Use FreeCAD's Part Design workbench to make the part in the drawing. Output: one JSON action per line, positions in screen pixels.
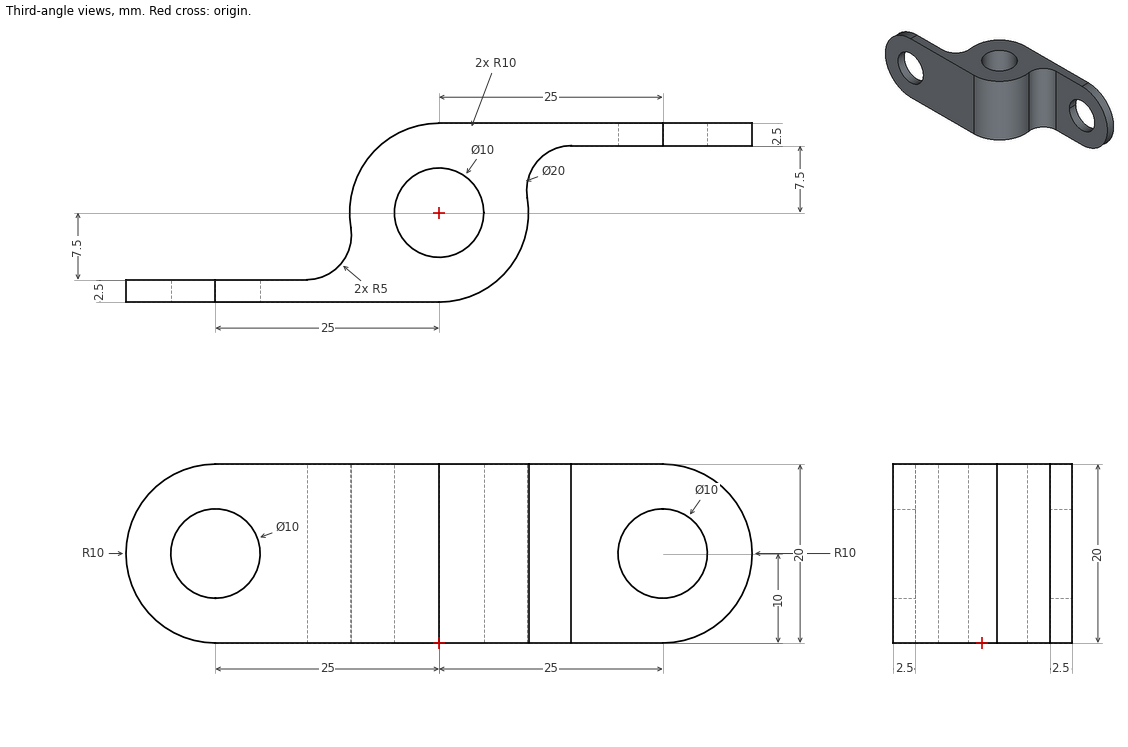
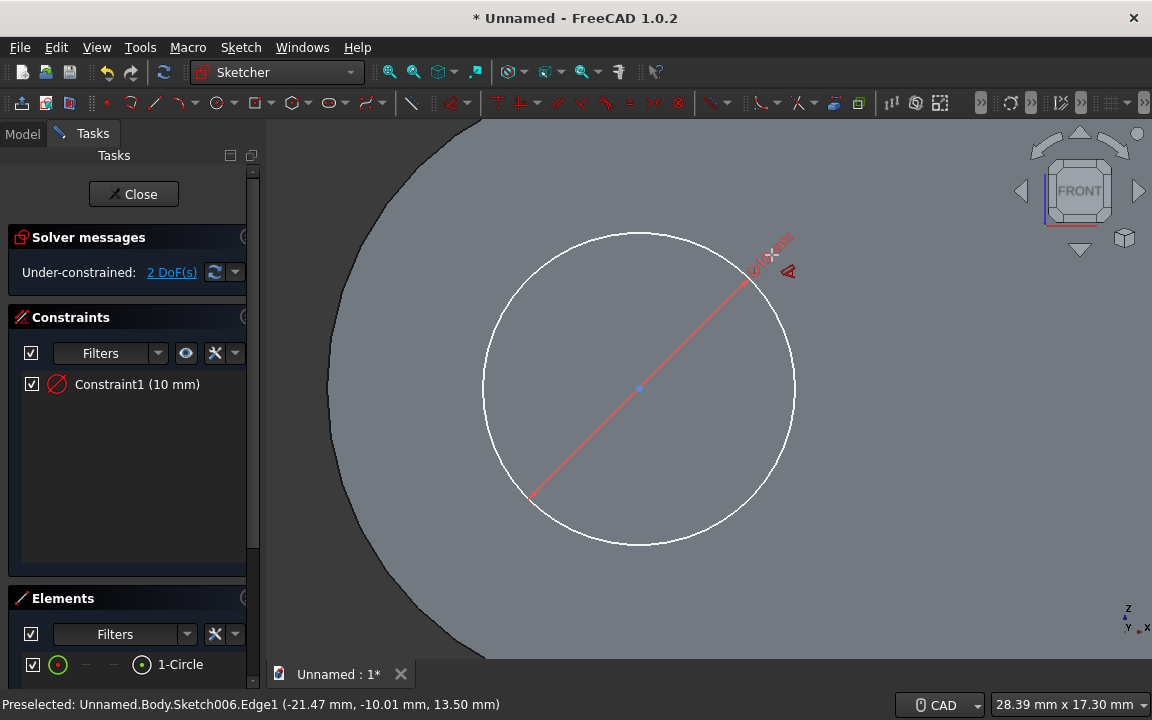
{"action": "left_click", "coordinate": [639, 389]}
{"action": "left_click", "coordinate": [813, 355]}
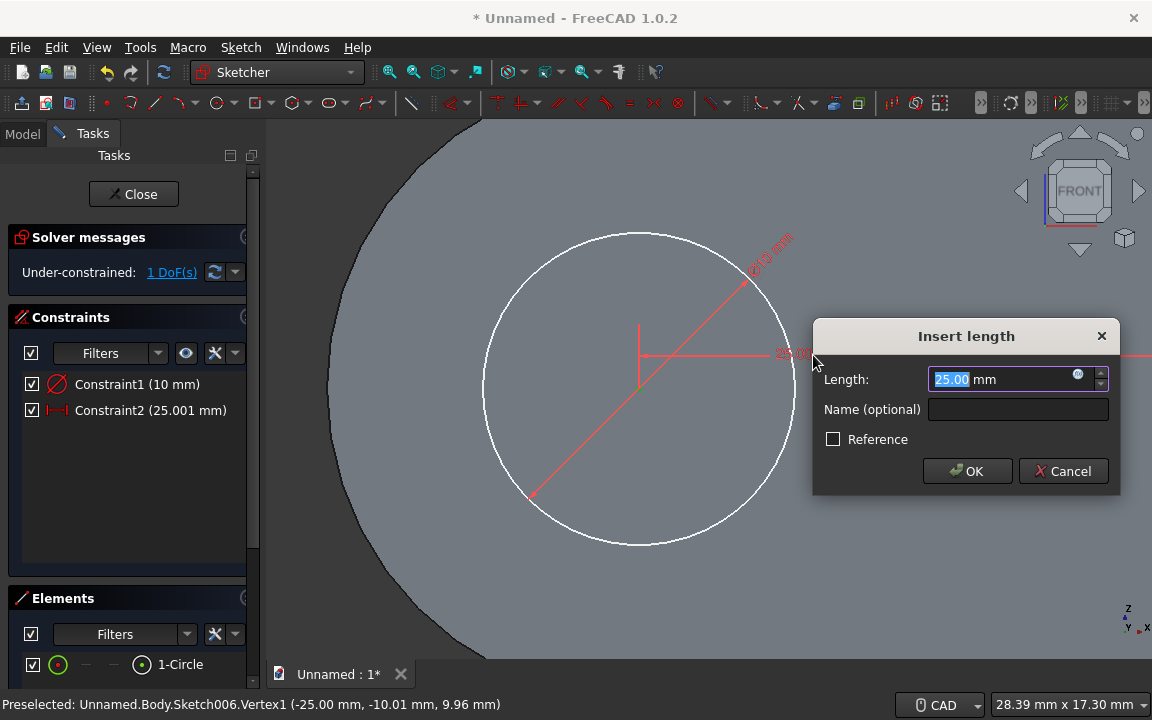
{"action": "type", "text": "25"}
{"action": "key", "text": "Return"}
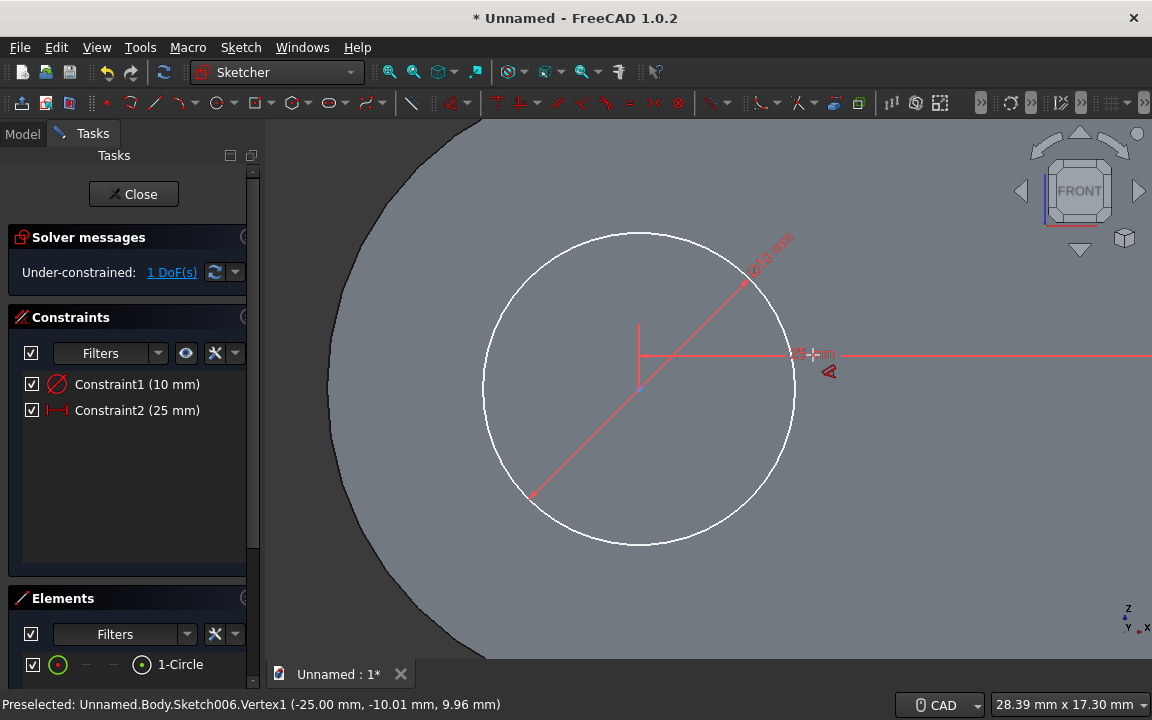
{"action": "left_click", "coordinate": [639, 389]}
{"action": "left_click", "coordinate": [605, 510]}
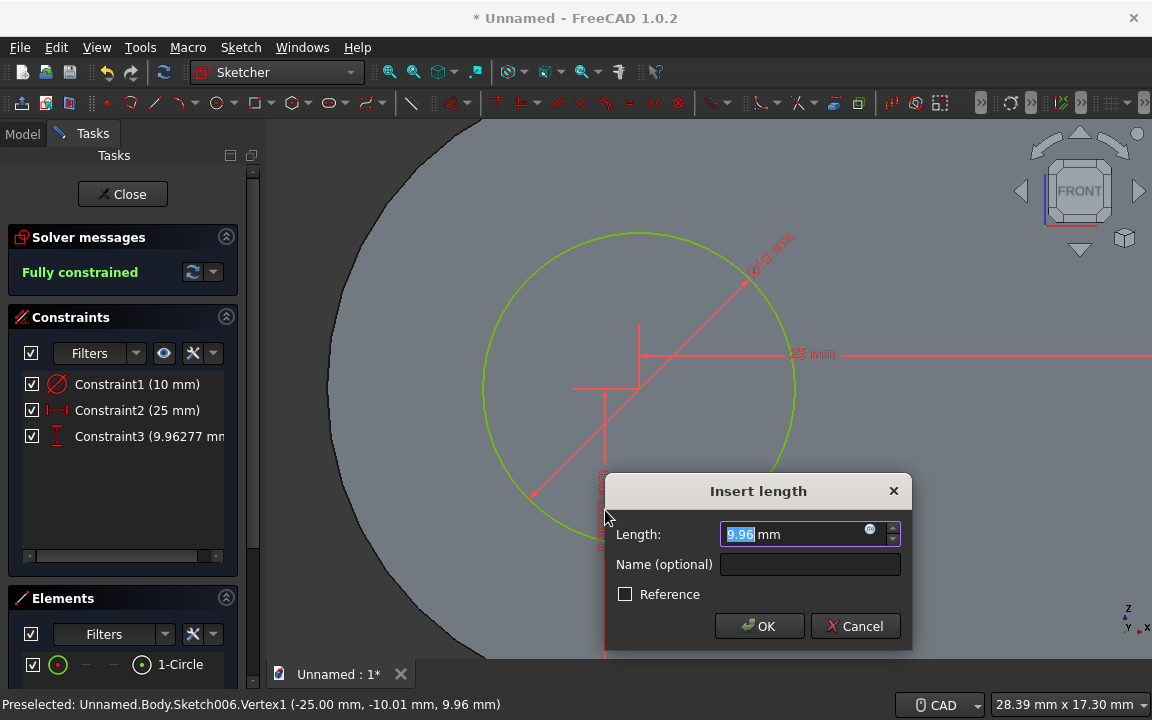
{"action": "type", "text": "10"}
{"action": "key", "text": "Return"}
{"action": "key", "text": "Escape"}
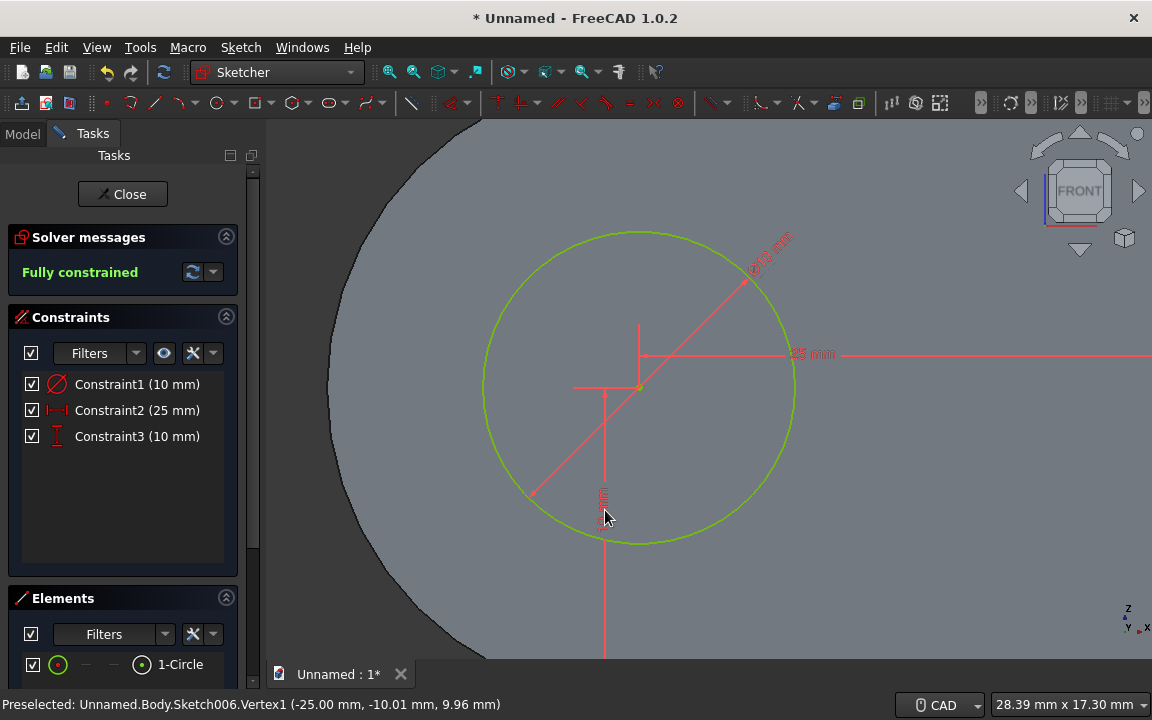
{"action": "left_click", "coordinate": [123, 194]}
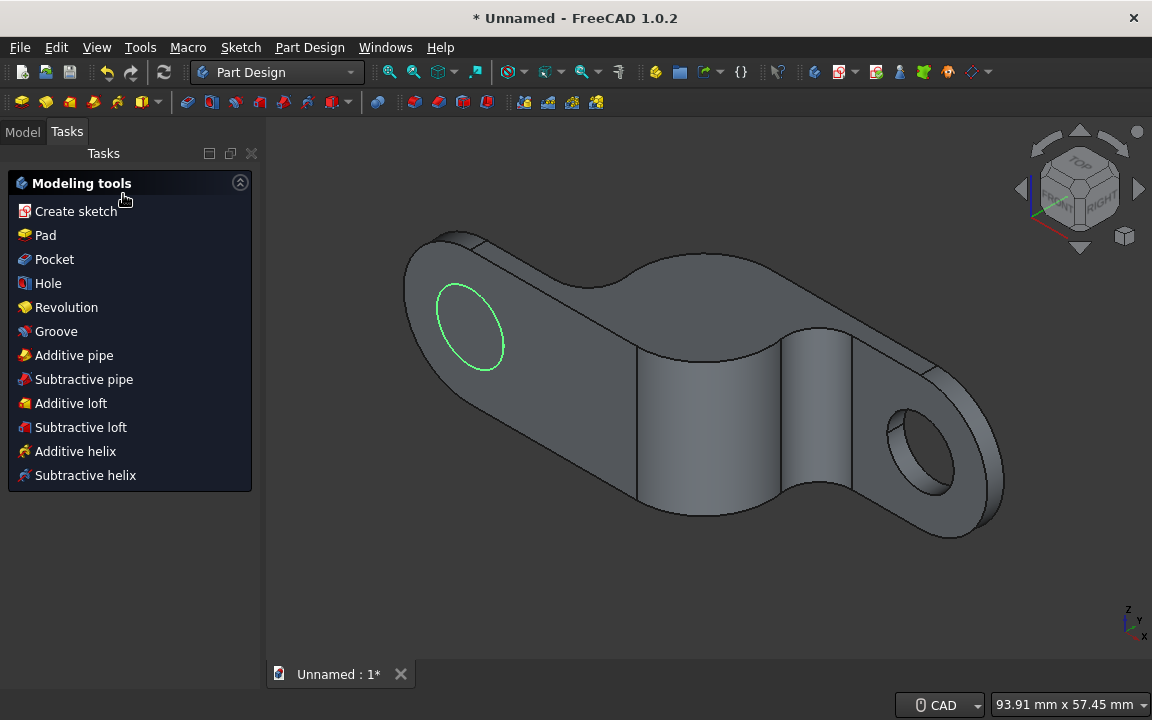
{"action": "left_click", "coordinate": [188, 102]}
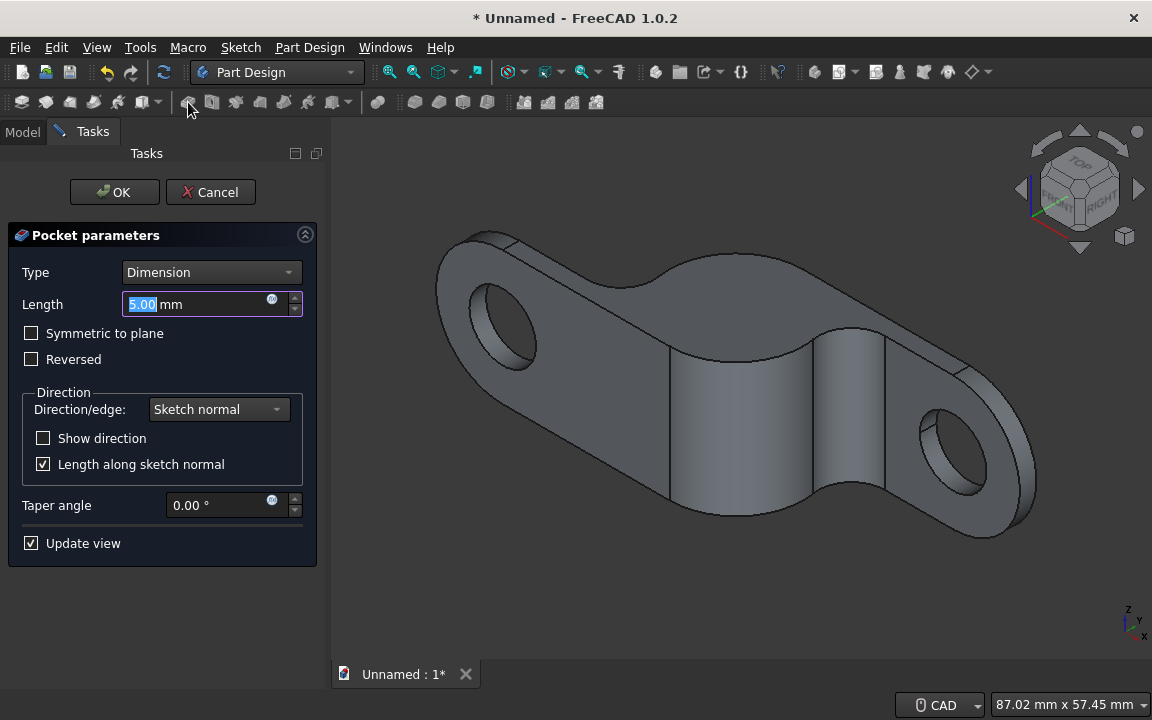
{"action": "type", "text": "2.5"}
{"action": "key", "text": "Tab"}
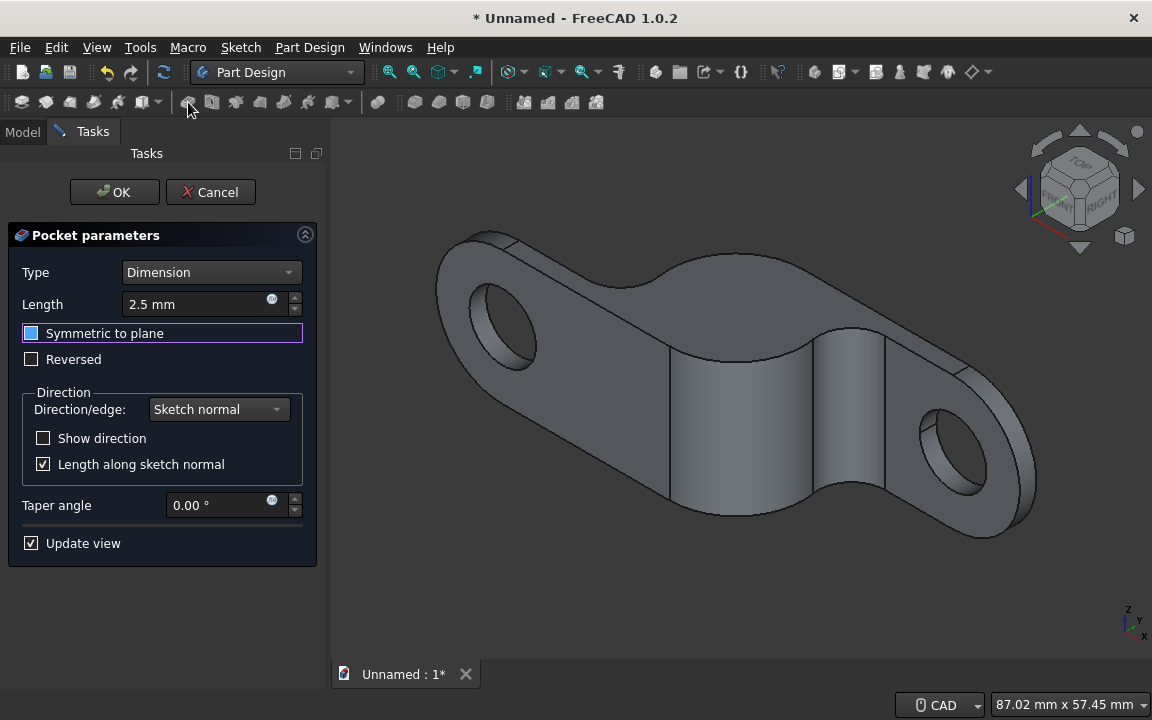
{"action": "left_click", "coordinate": [115, 192]}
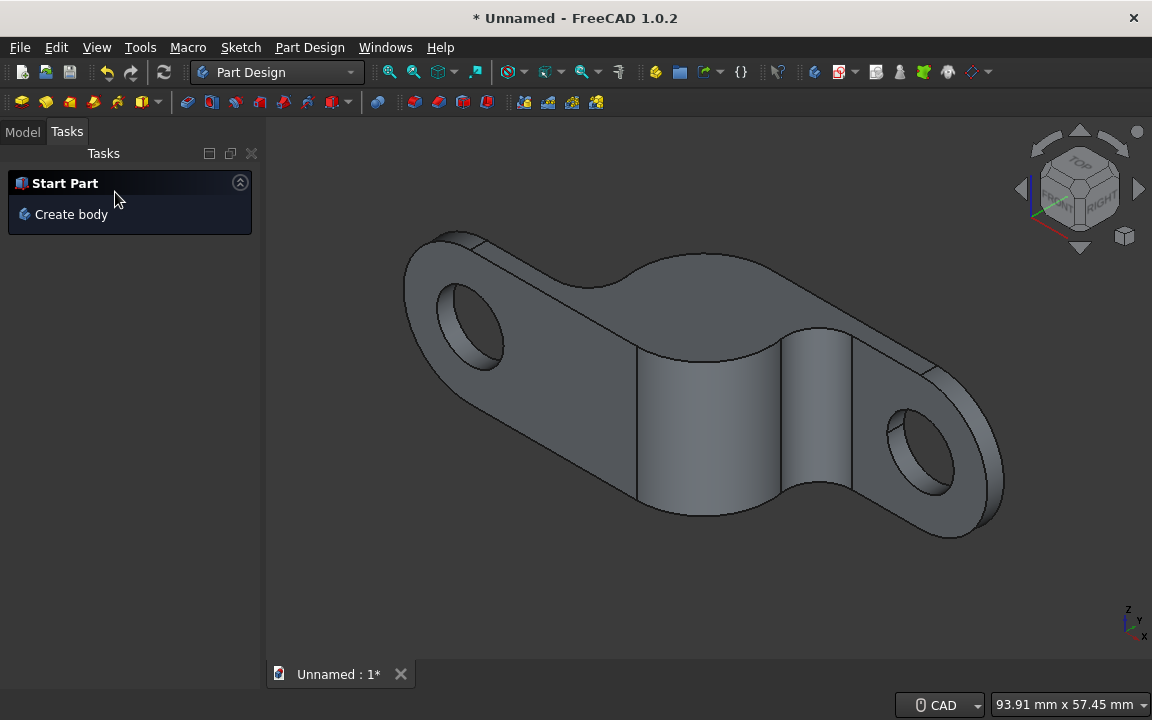
{"action": "left_click", "coordinate": [704, 307]}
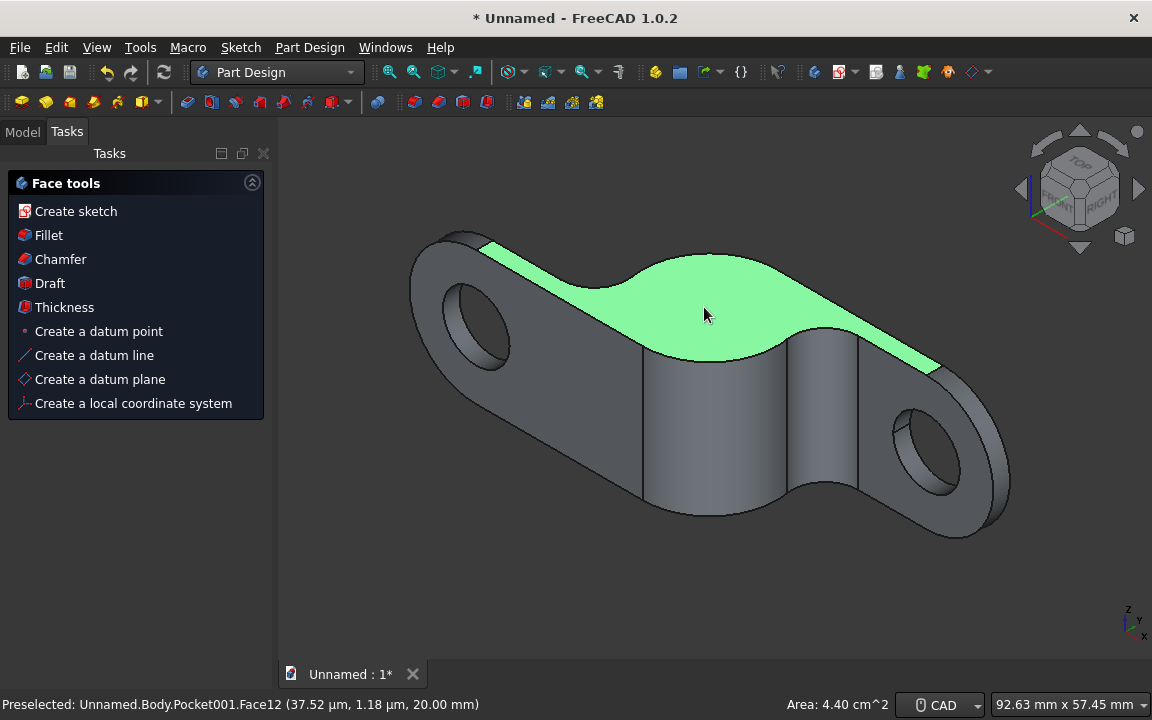
{"action": "left_click", "coordinate": [840, 72]}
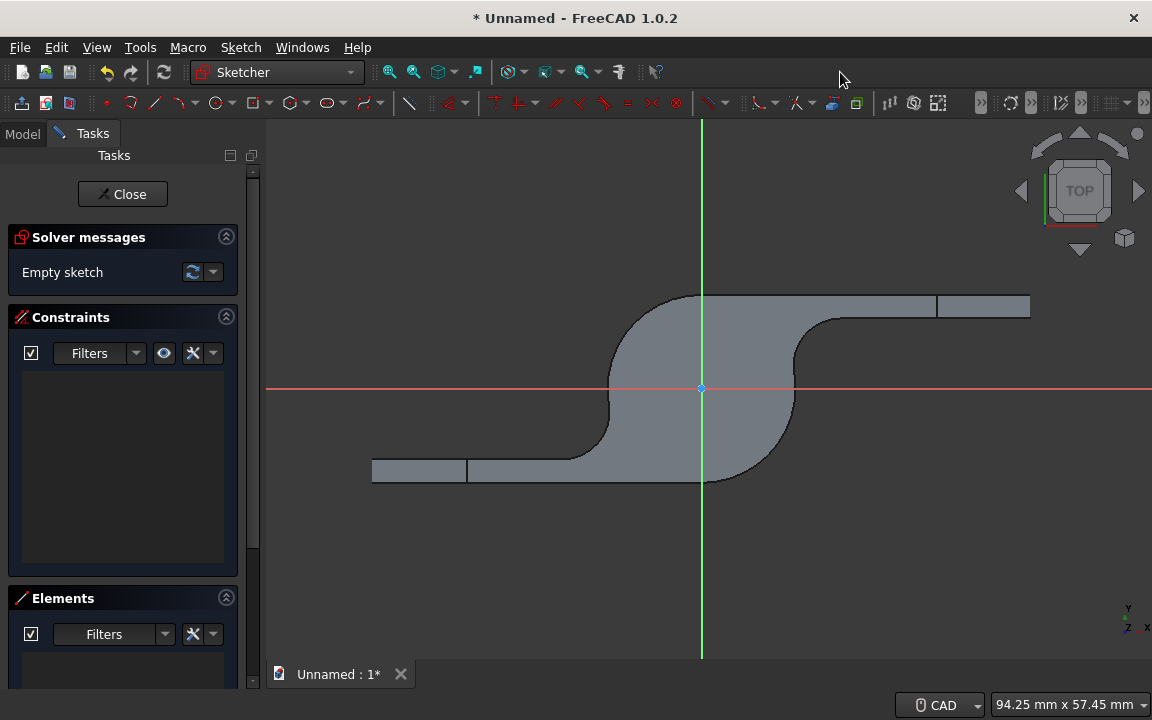
{"action": "scroll", "coordinate": [728, 389], "scroll_direction": "up", "scroll_amount": 6}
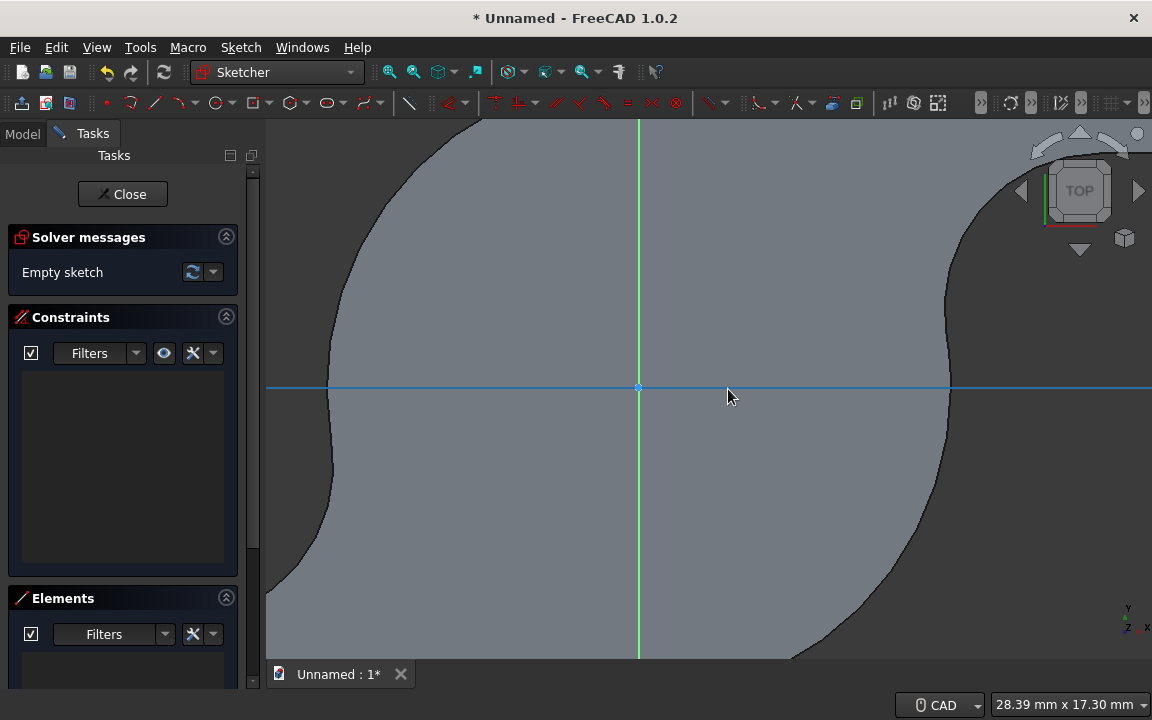
{"action": "key", "text": "g c"}